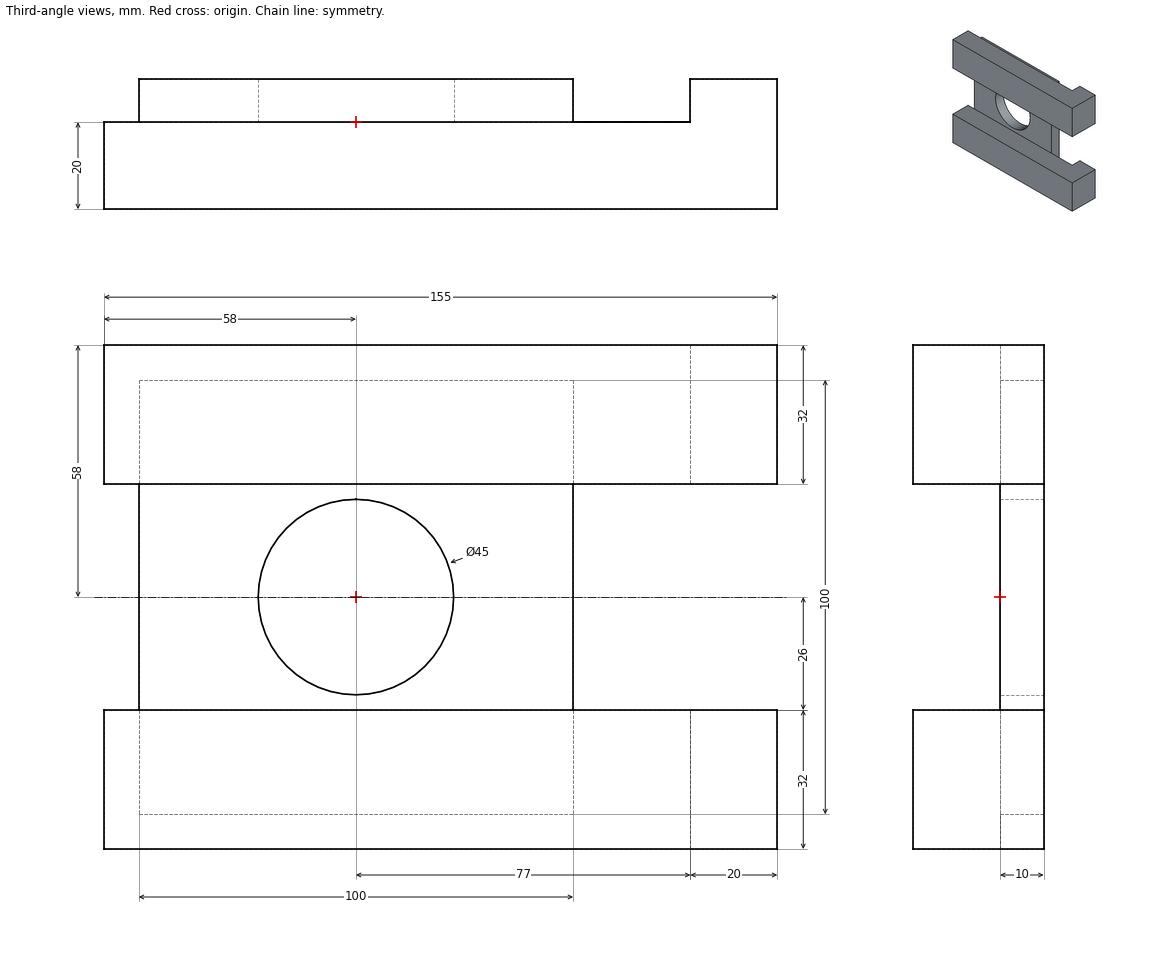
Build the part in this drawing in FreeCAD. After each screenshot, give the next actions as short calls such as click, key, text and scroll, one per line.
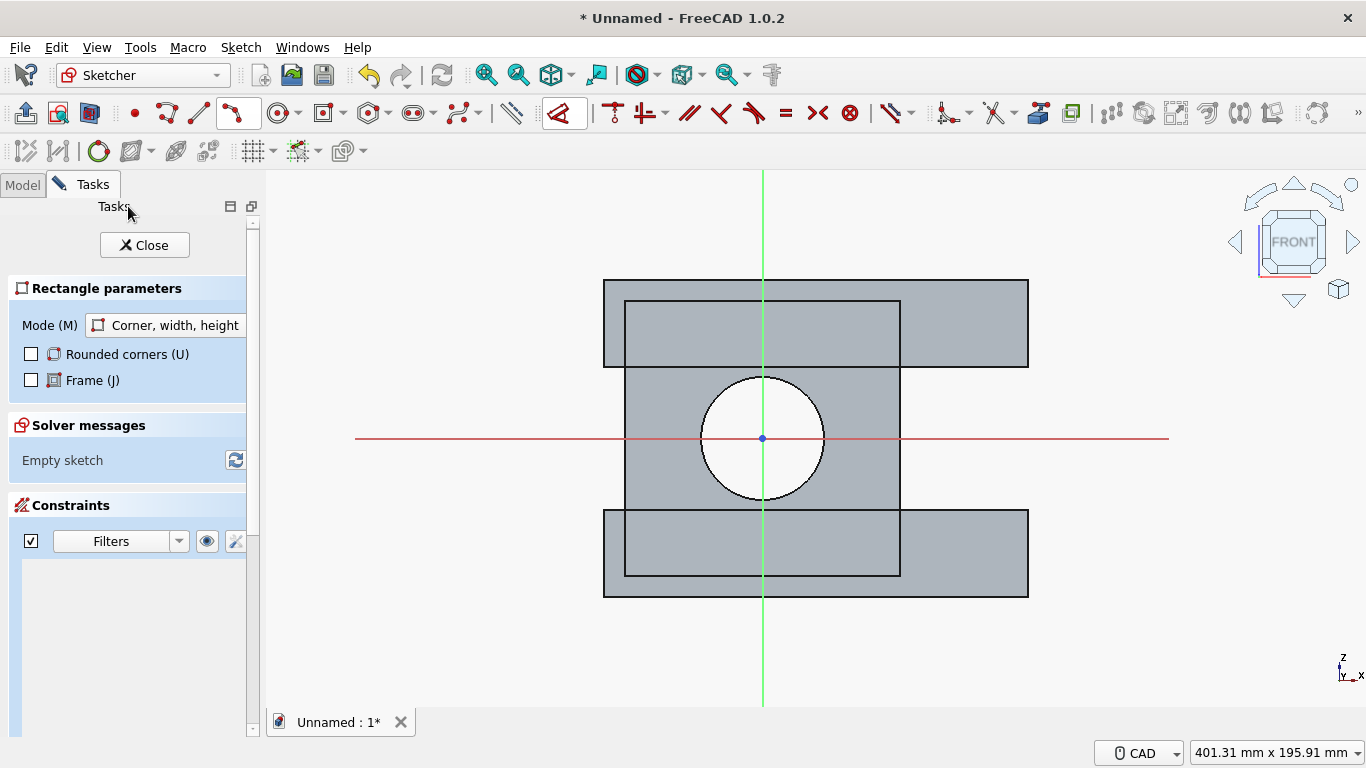
click(974, 510)
move(1028, 597)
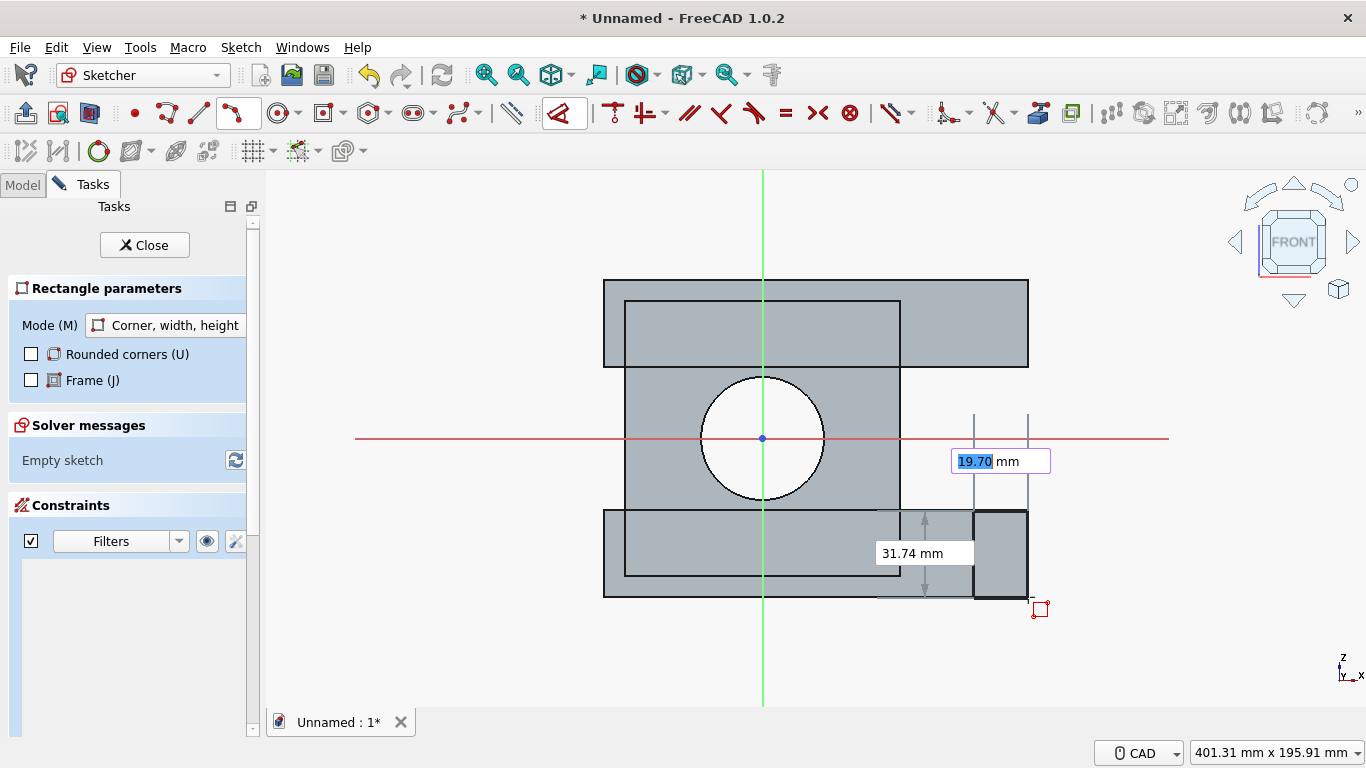
text(20)
key(Tab)
text(32)
key(Return)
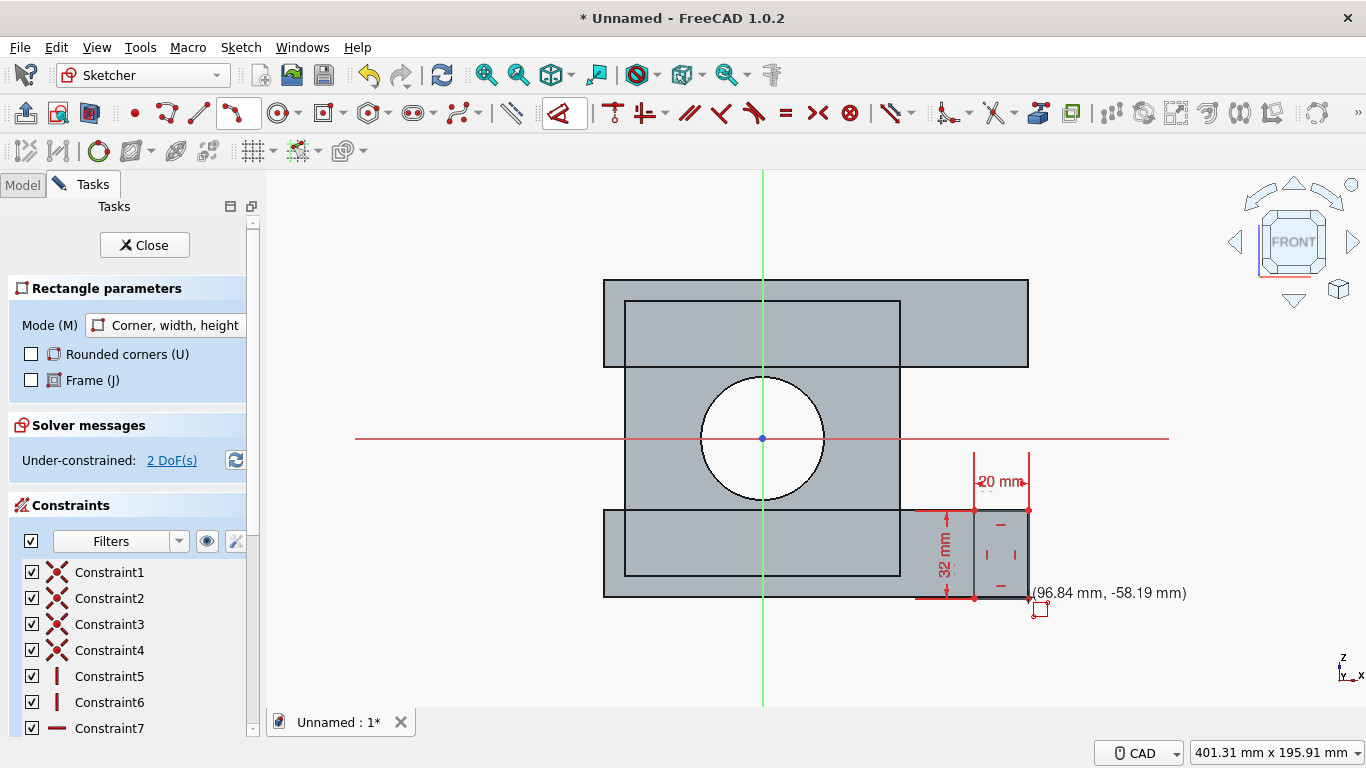
click(974, 280)
move(1028, 367)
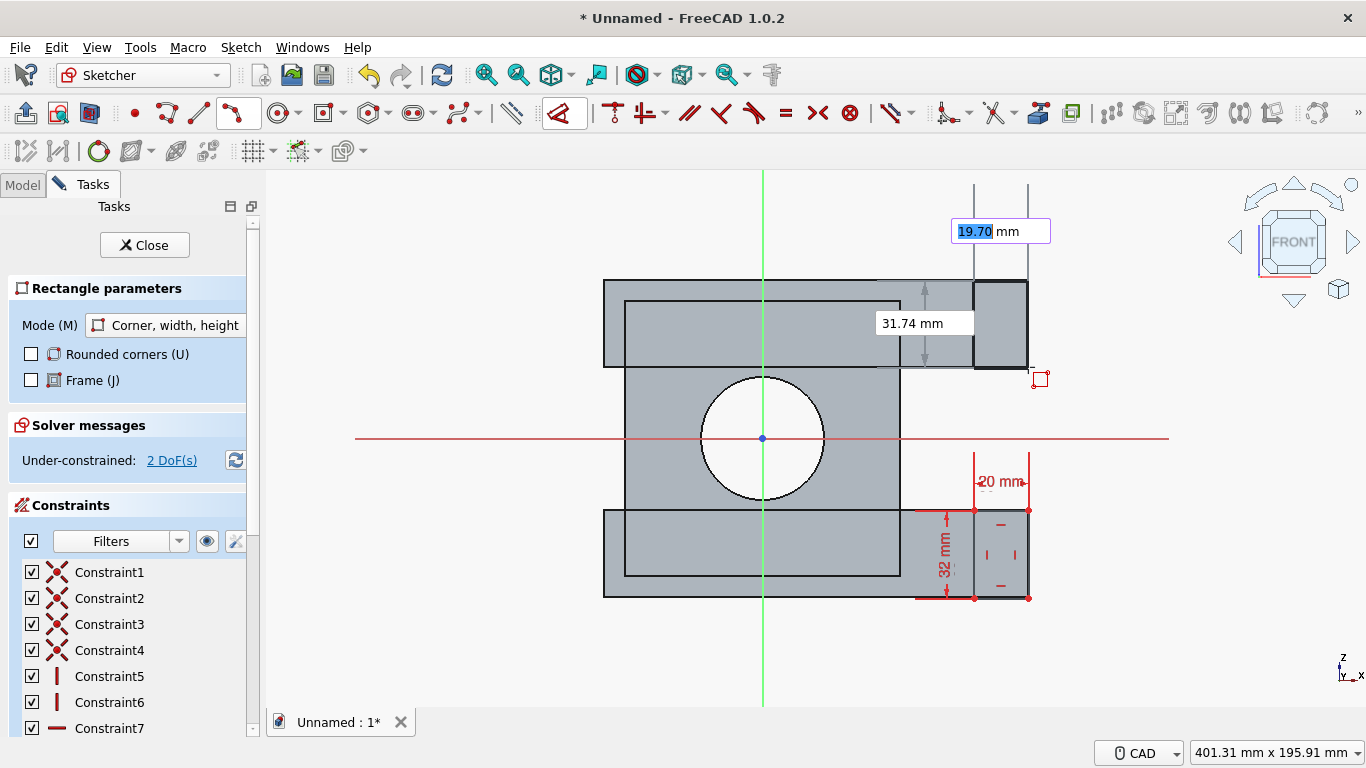
text(20)
key(Tab)
text(32)
key(Return)
key(Escape)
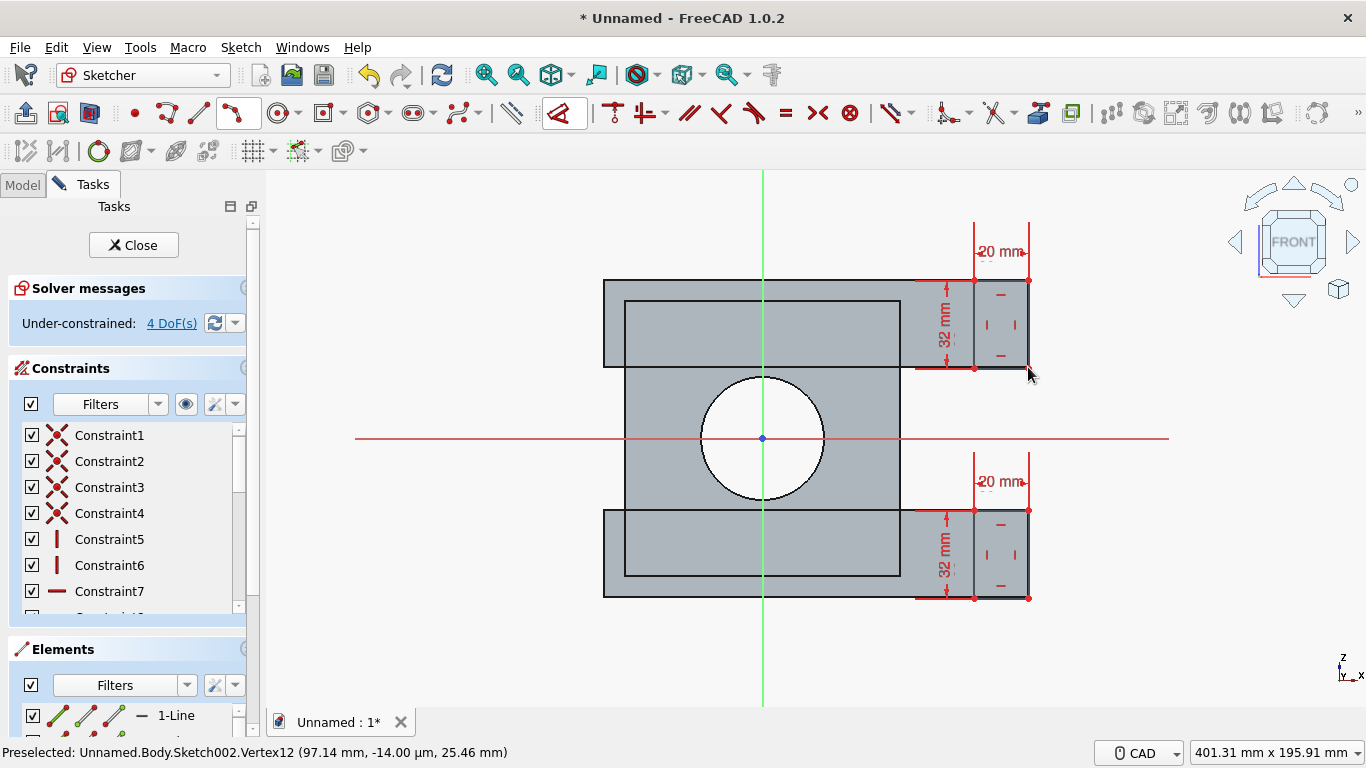
click(974, 599)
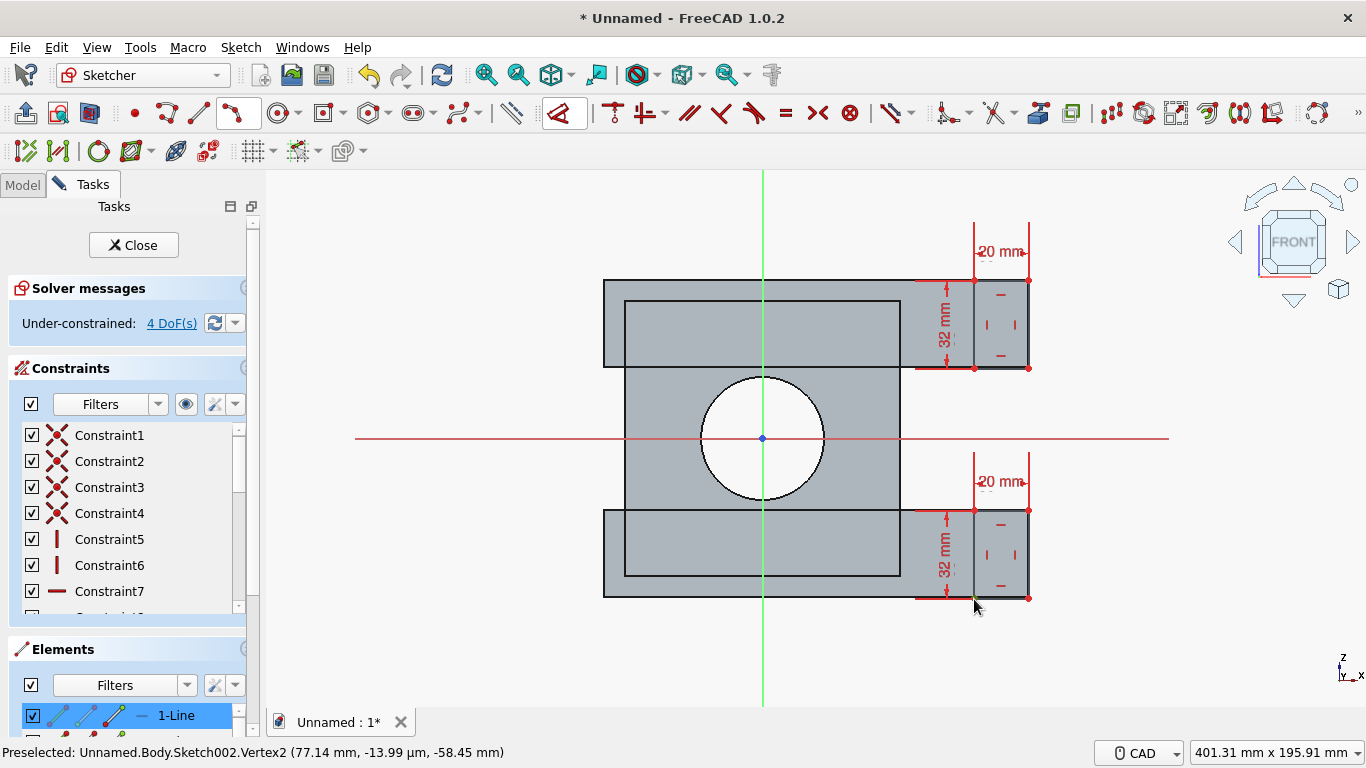
click(974, 281)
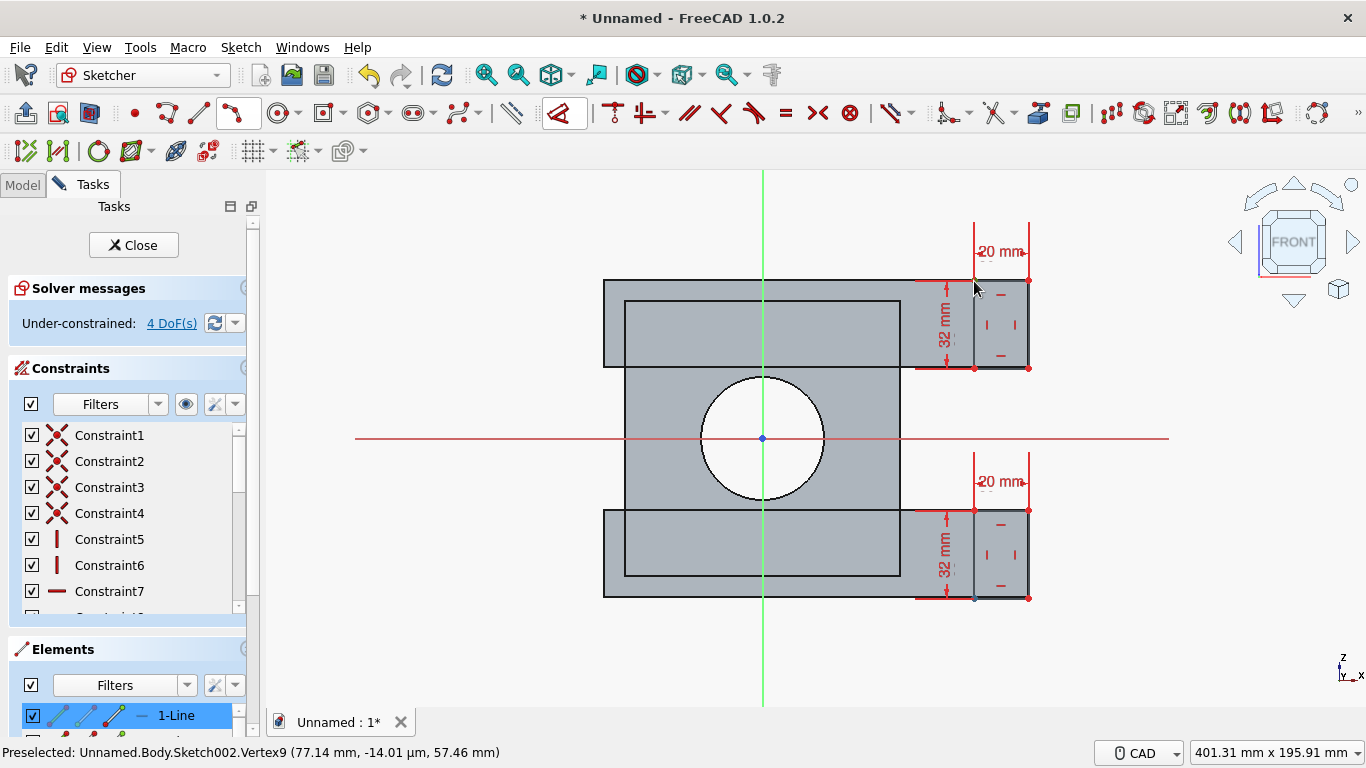
click(359, 438)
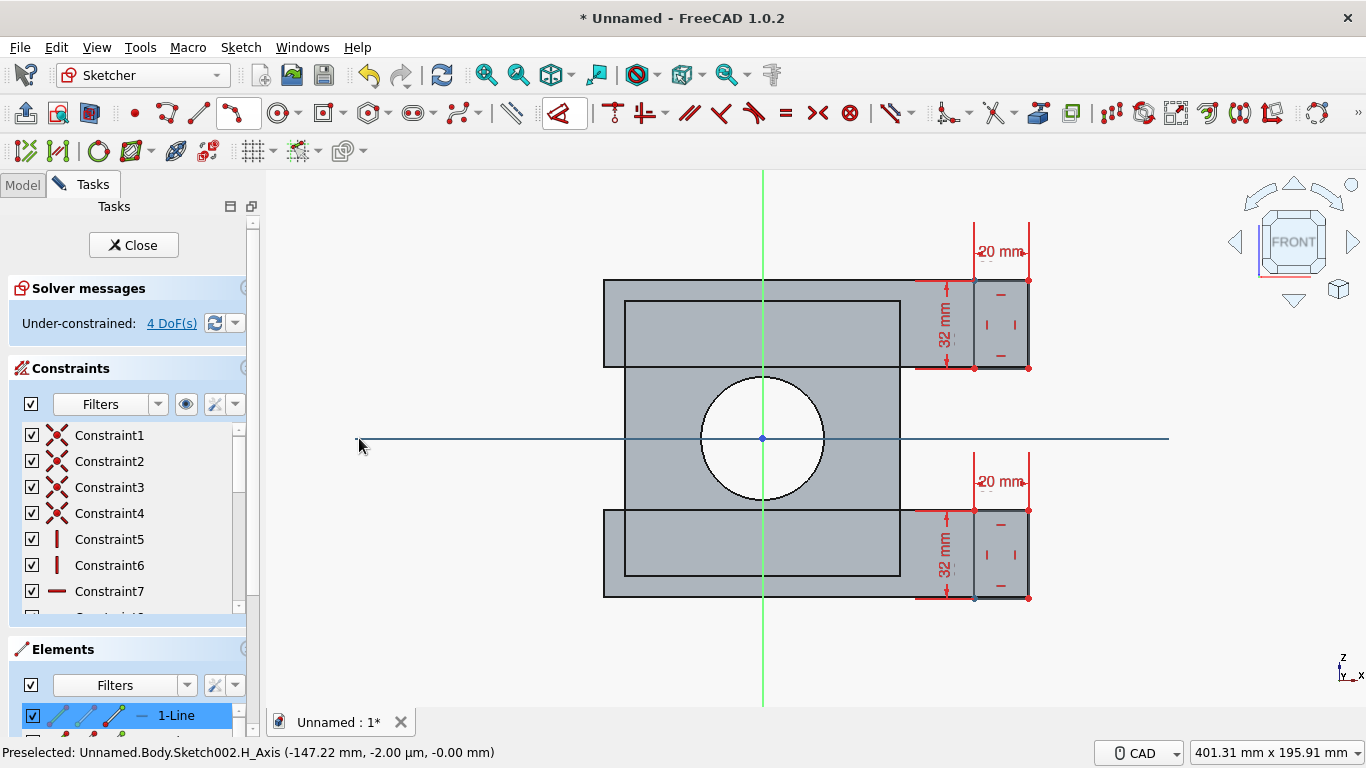
key(s)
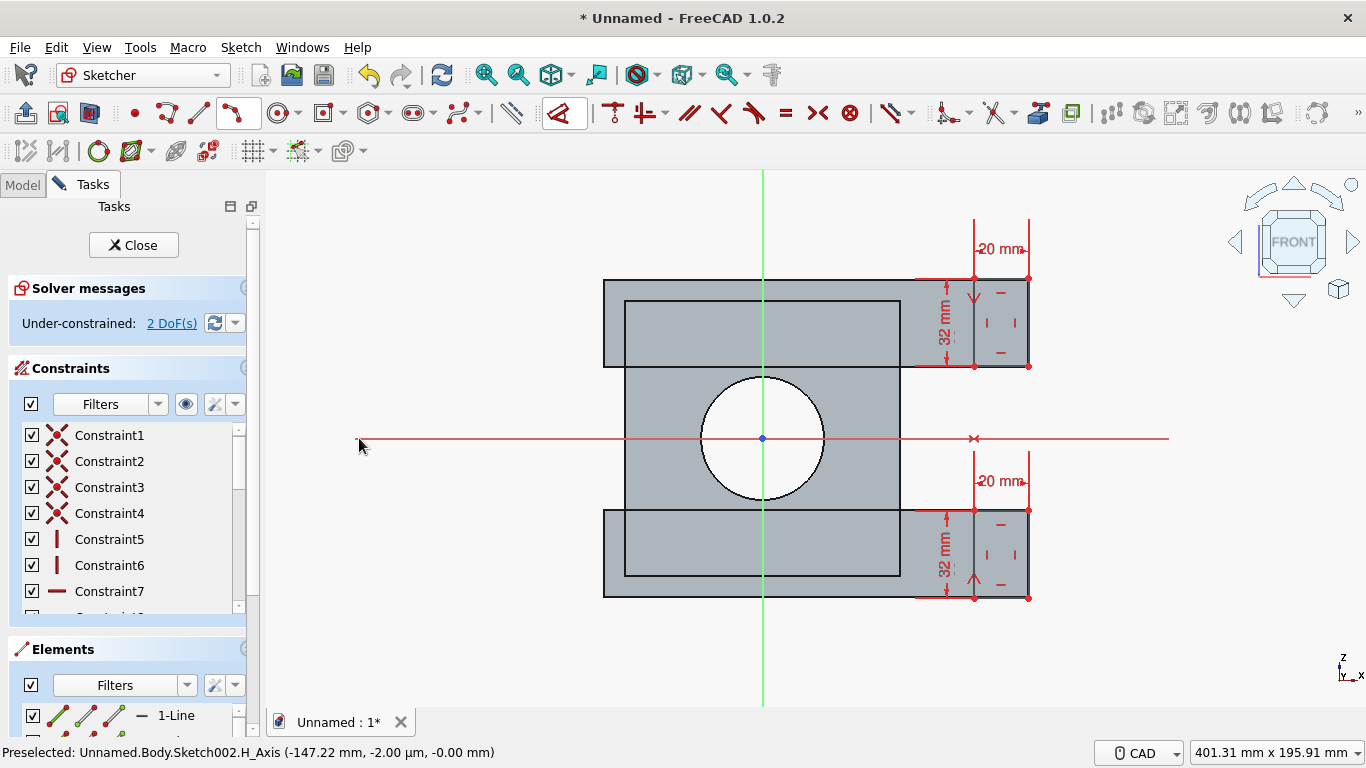
key(d)